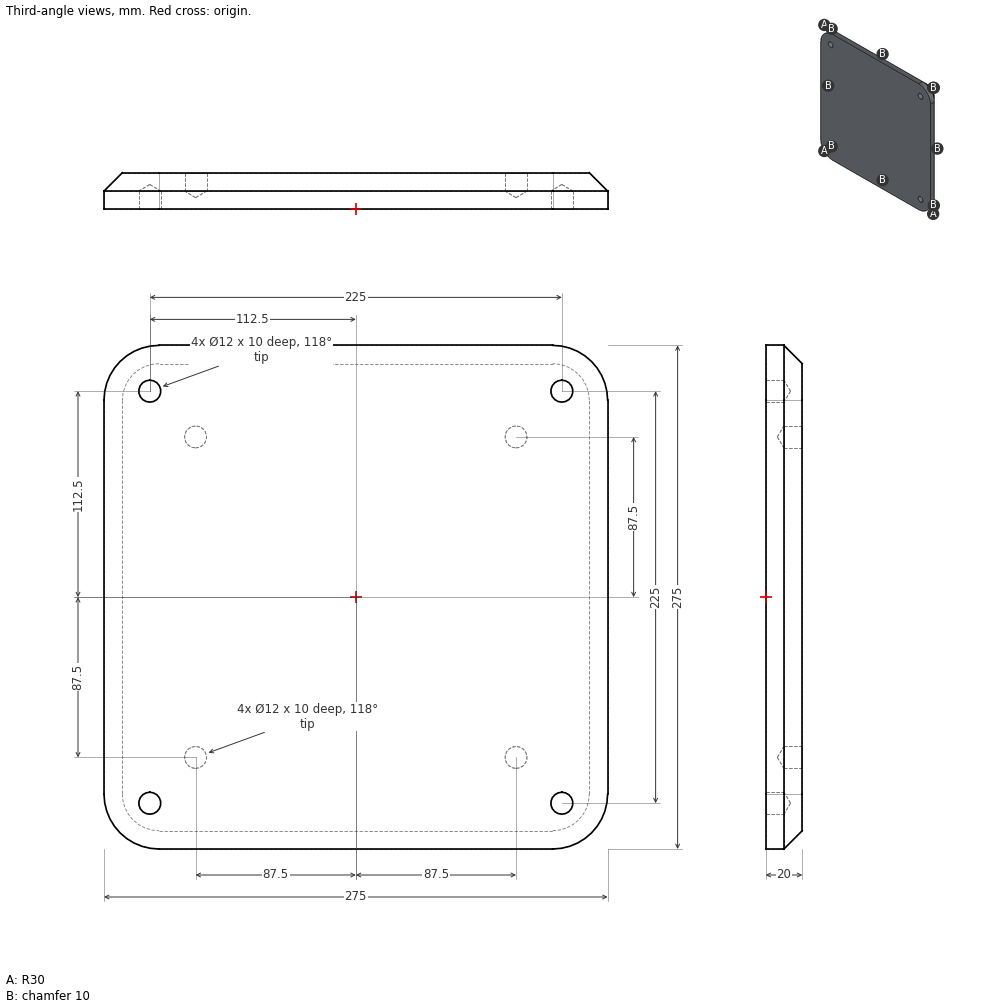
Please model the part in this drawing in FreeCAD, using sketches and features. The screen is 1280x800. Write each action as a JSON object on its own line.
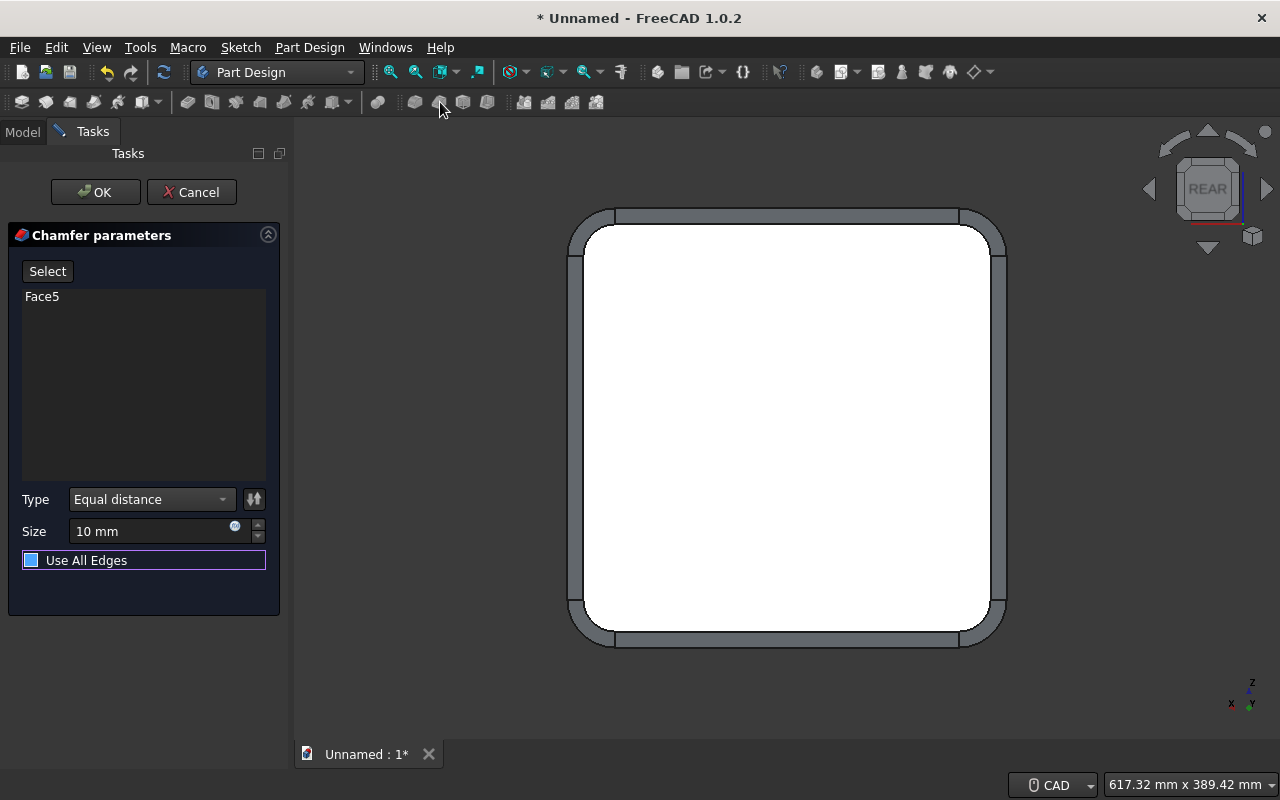
{"action": "left_click", "coordinate": [96, 192]}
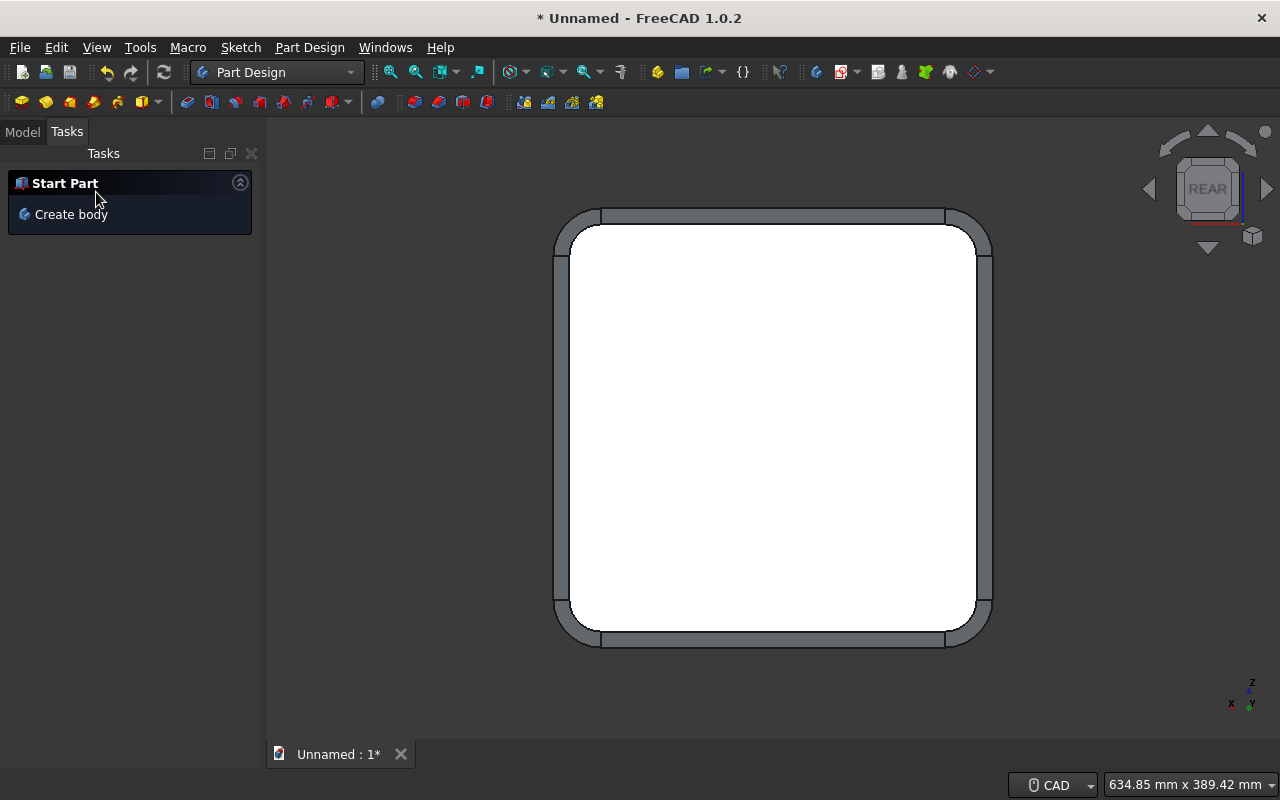
{"action": "left_click", "coordinate": [773, 427]}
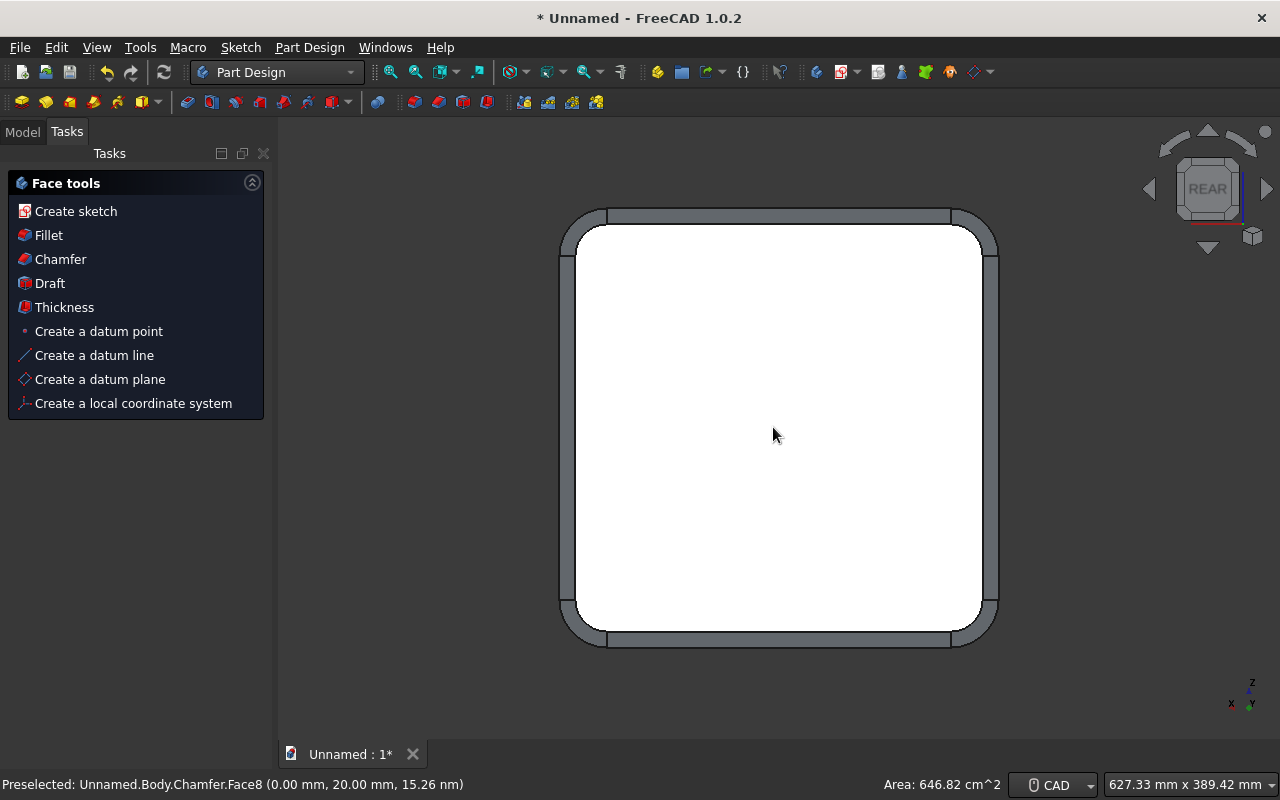
{"action": "left_click", "coordinate": [842, 72]}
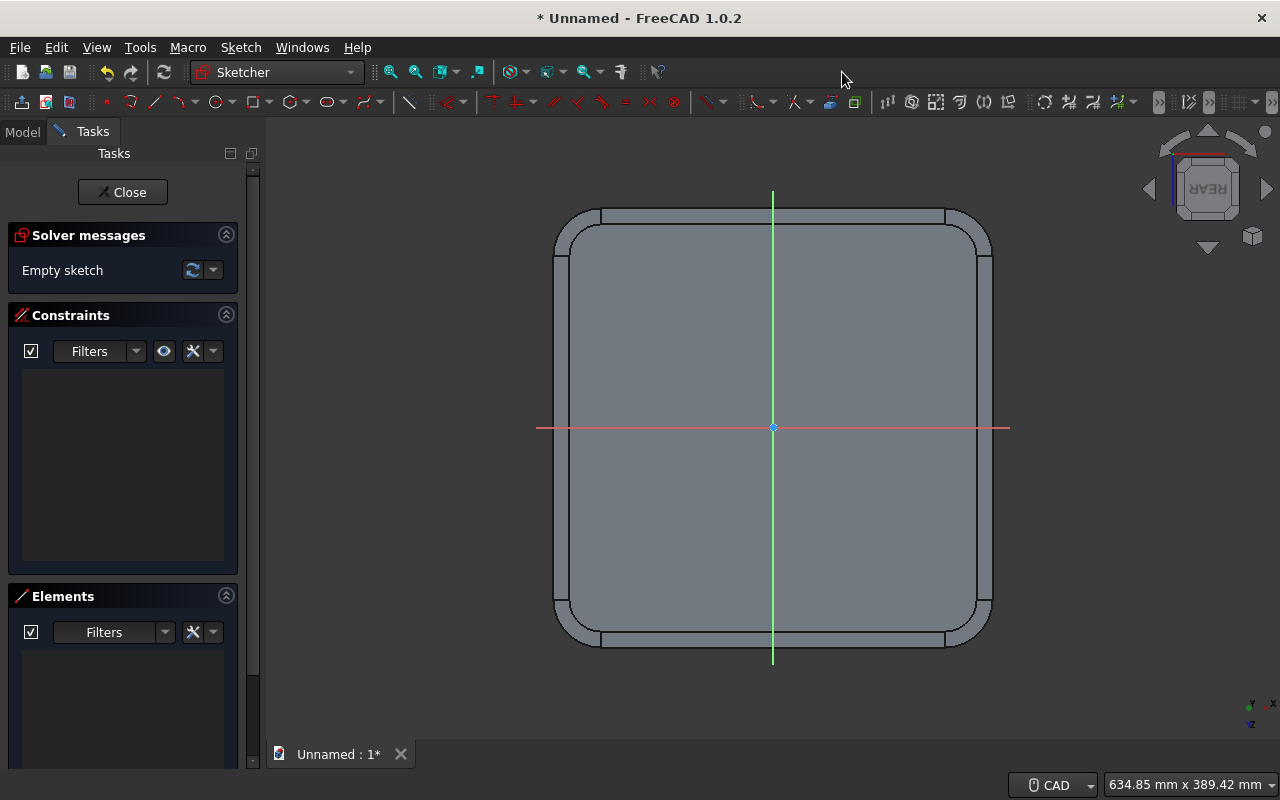
{"action": "key", "text": "g c"}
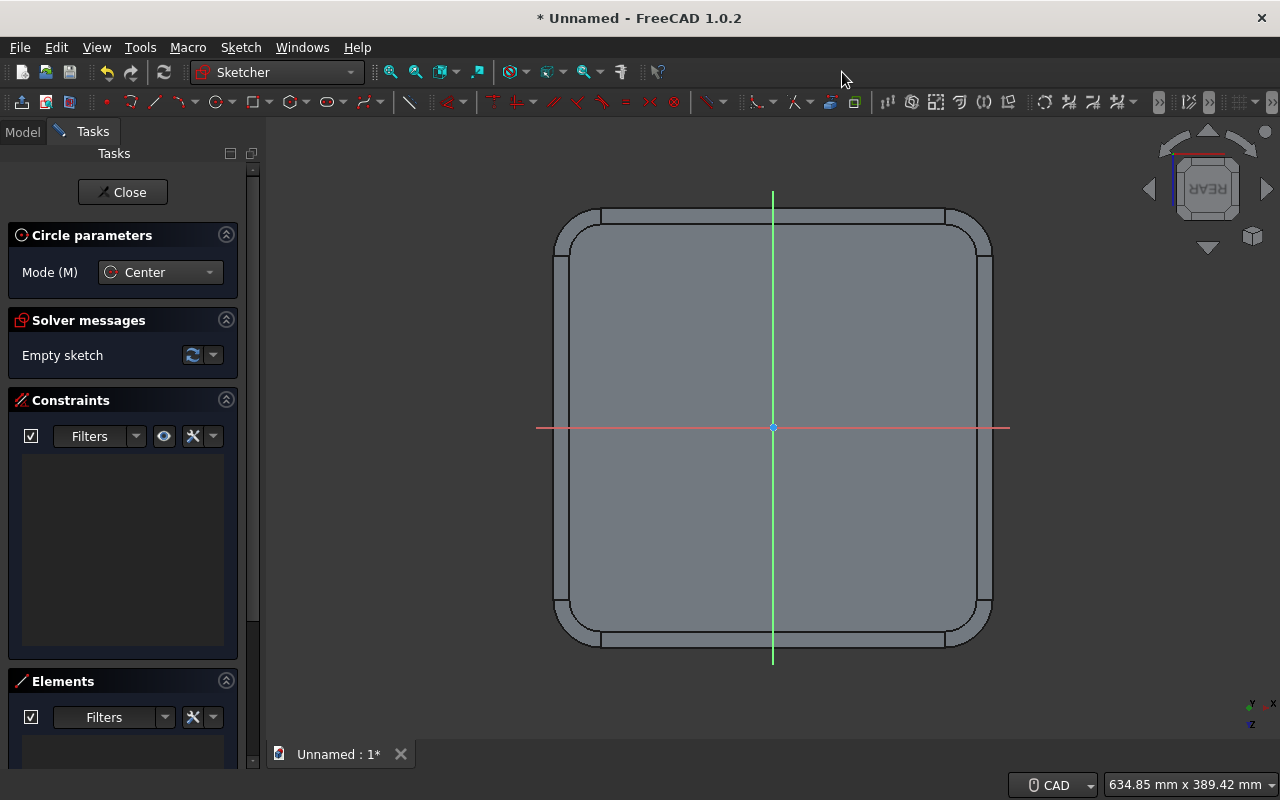
{"action": "scroll", "coordinate": [633, 288], "scroll_direction": "up", "scroll_amount": 5}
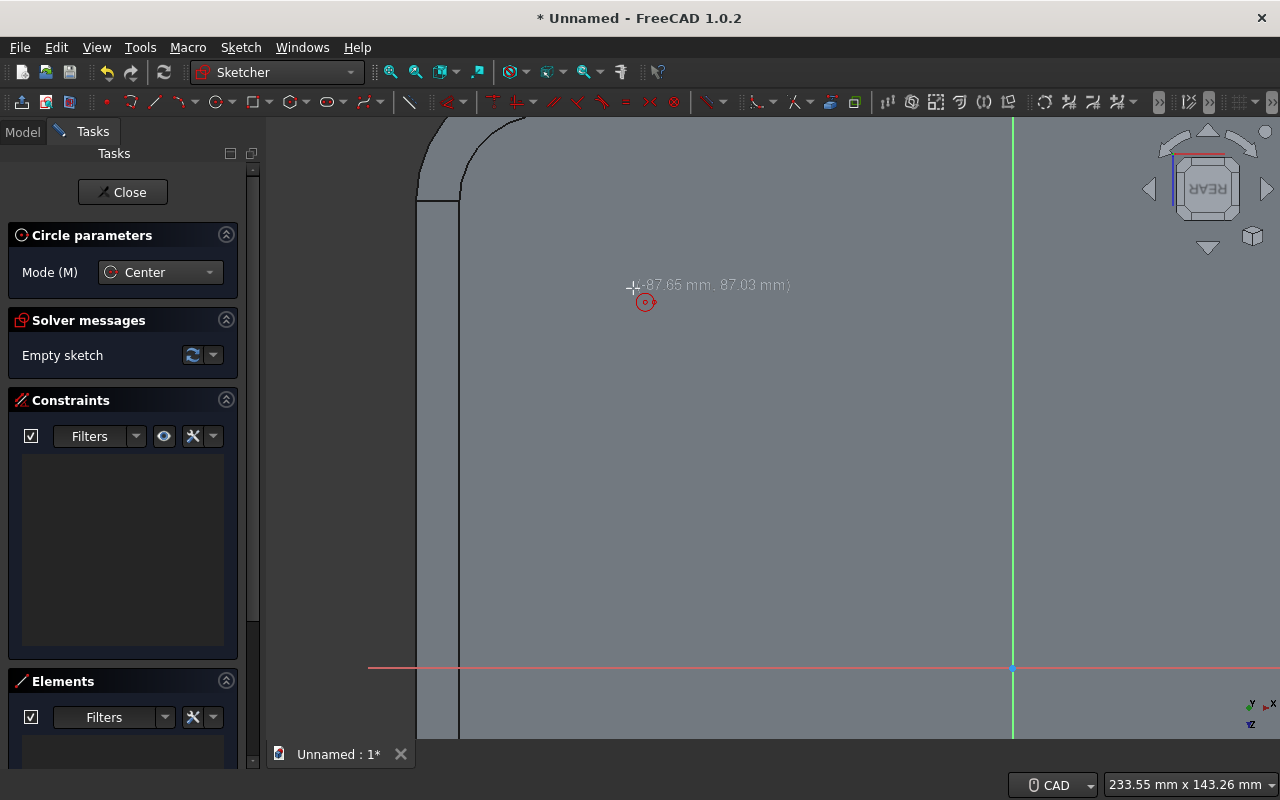
{"action": "left_click", "coordinate": [633, 288]}
{"action": "mouse_move", "coordinate": [651, 270]}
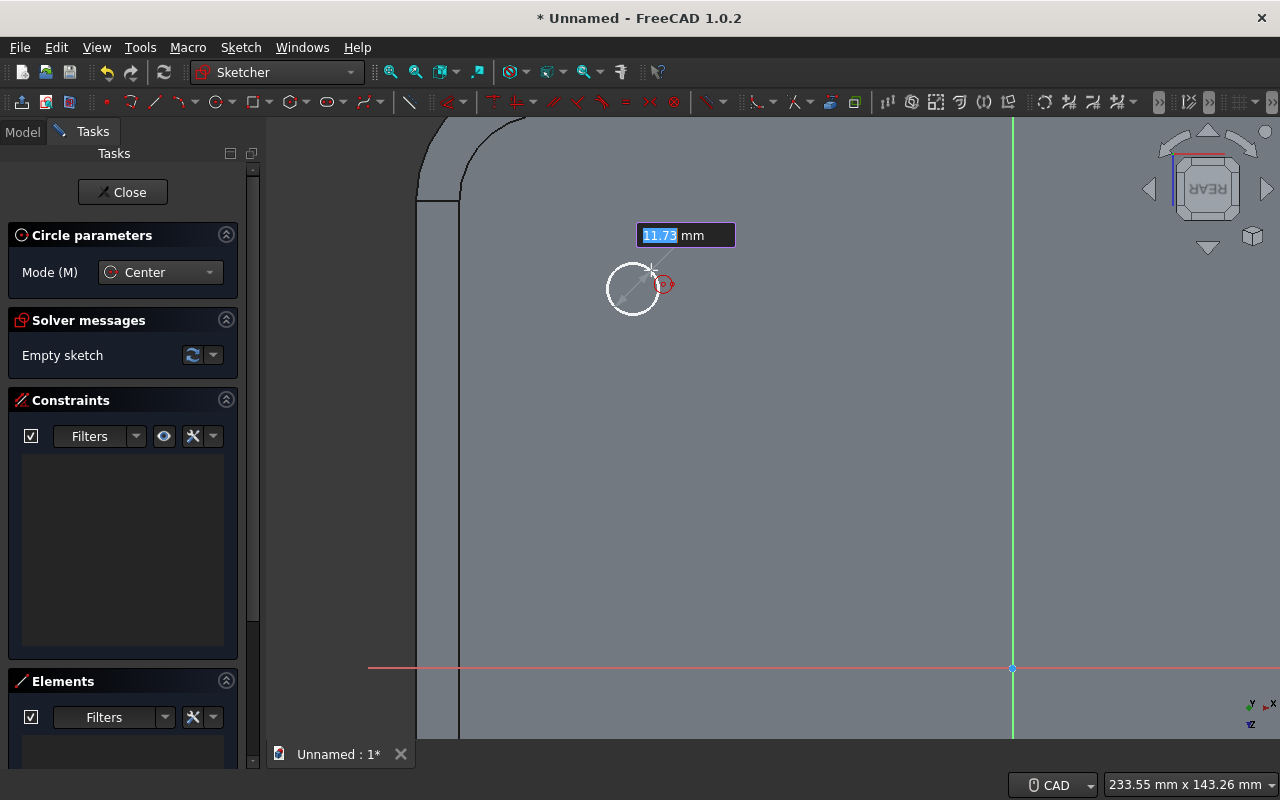
{"action": "type", "text": "12"}
{"action": "key", "text": "Return"}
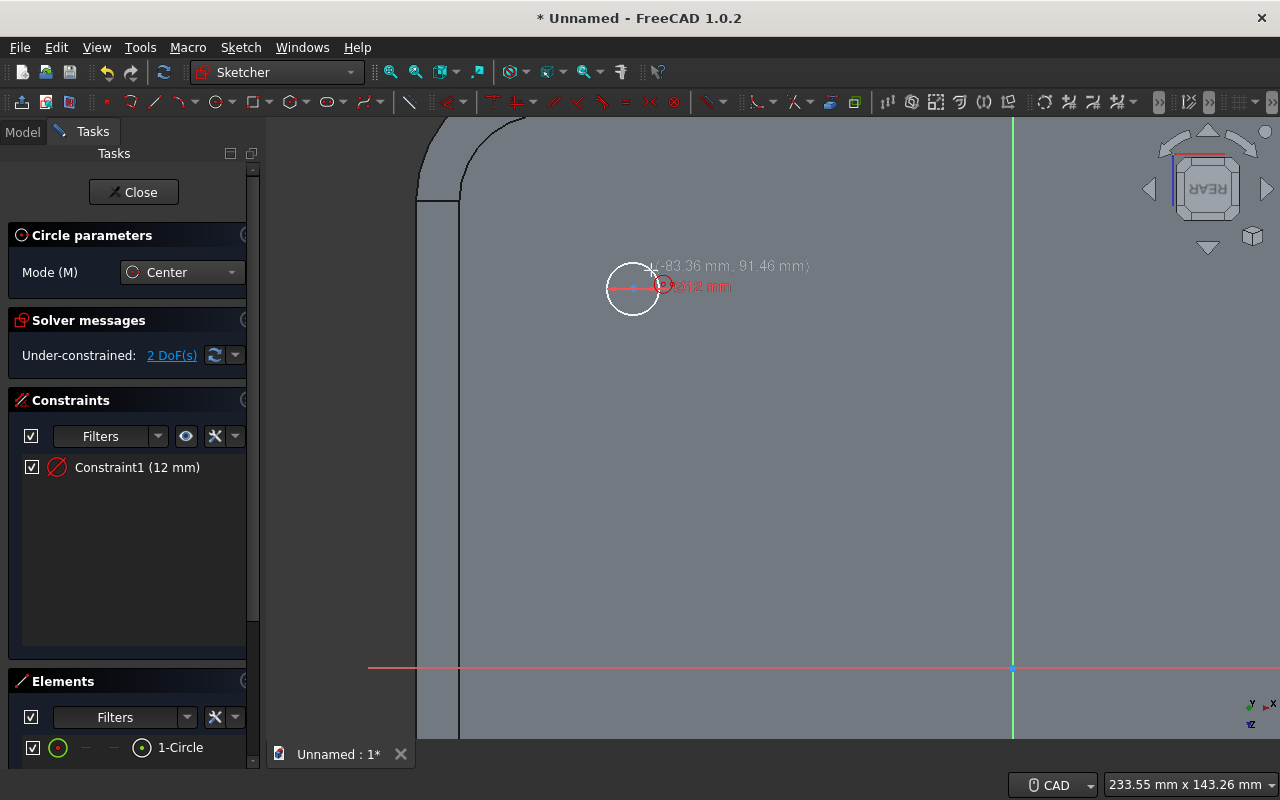
{"action": "scroll", "coordinate": [453, 232], "scroll_direction": "down", "scroll_amount": 4}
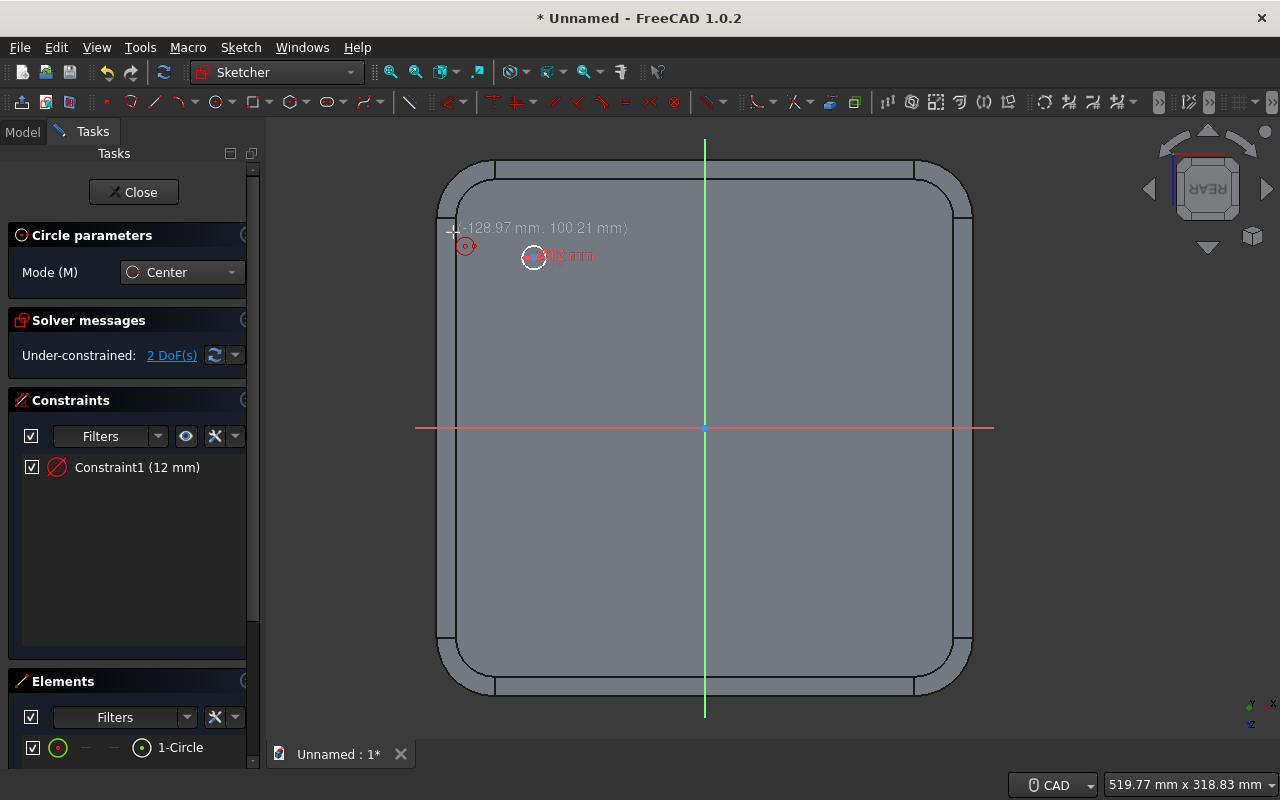
{"action": "scroll", "coordinate": [875, 257], "scroll_direction": "up", "scroll_amount": 4}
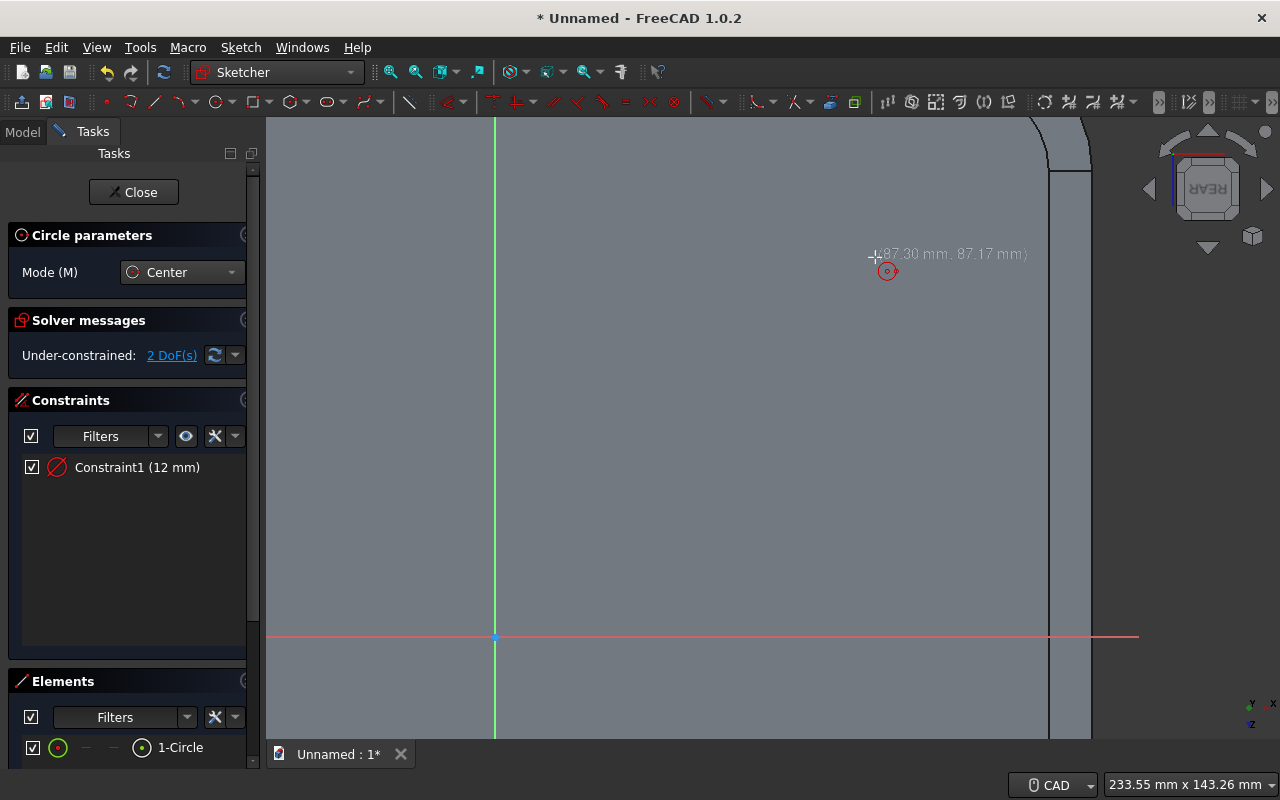
{"action": "left_click", "coordinate": [875, 257]}
{"action": "mouse_move", "coordinate": [894, 239]}